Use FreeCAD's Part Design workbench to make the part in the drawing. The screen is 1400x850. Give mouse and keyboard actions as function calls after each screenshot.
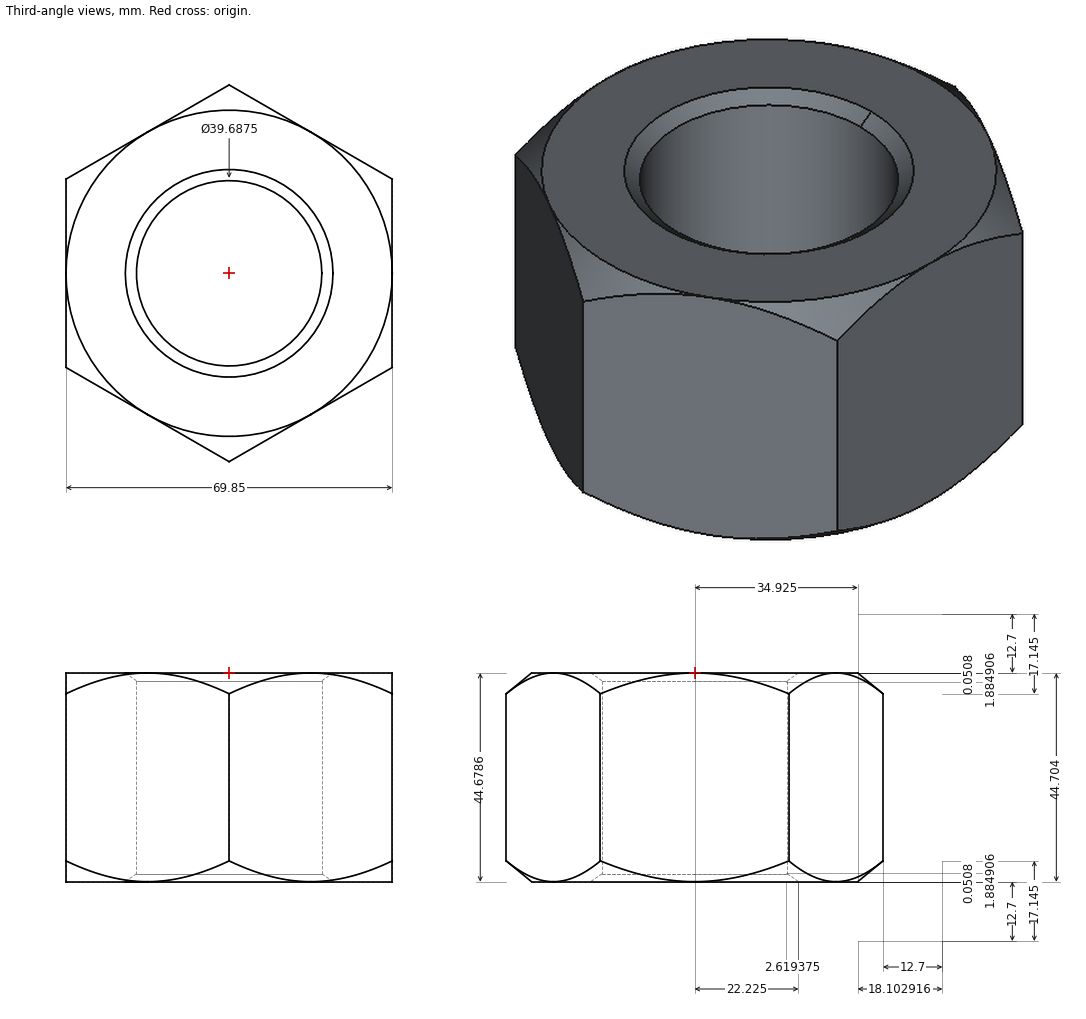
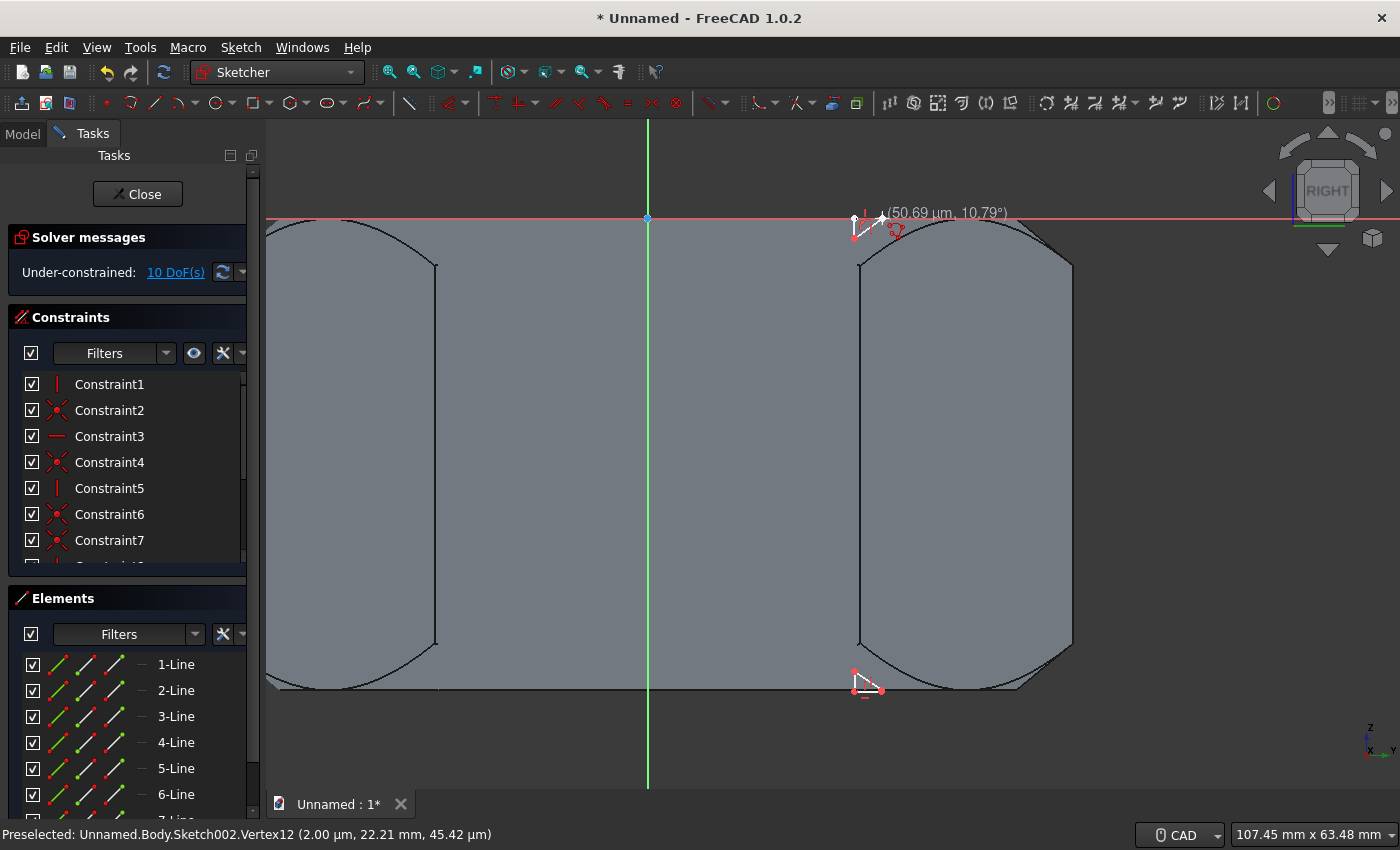
scroll(855, 218, up, 17)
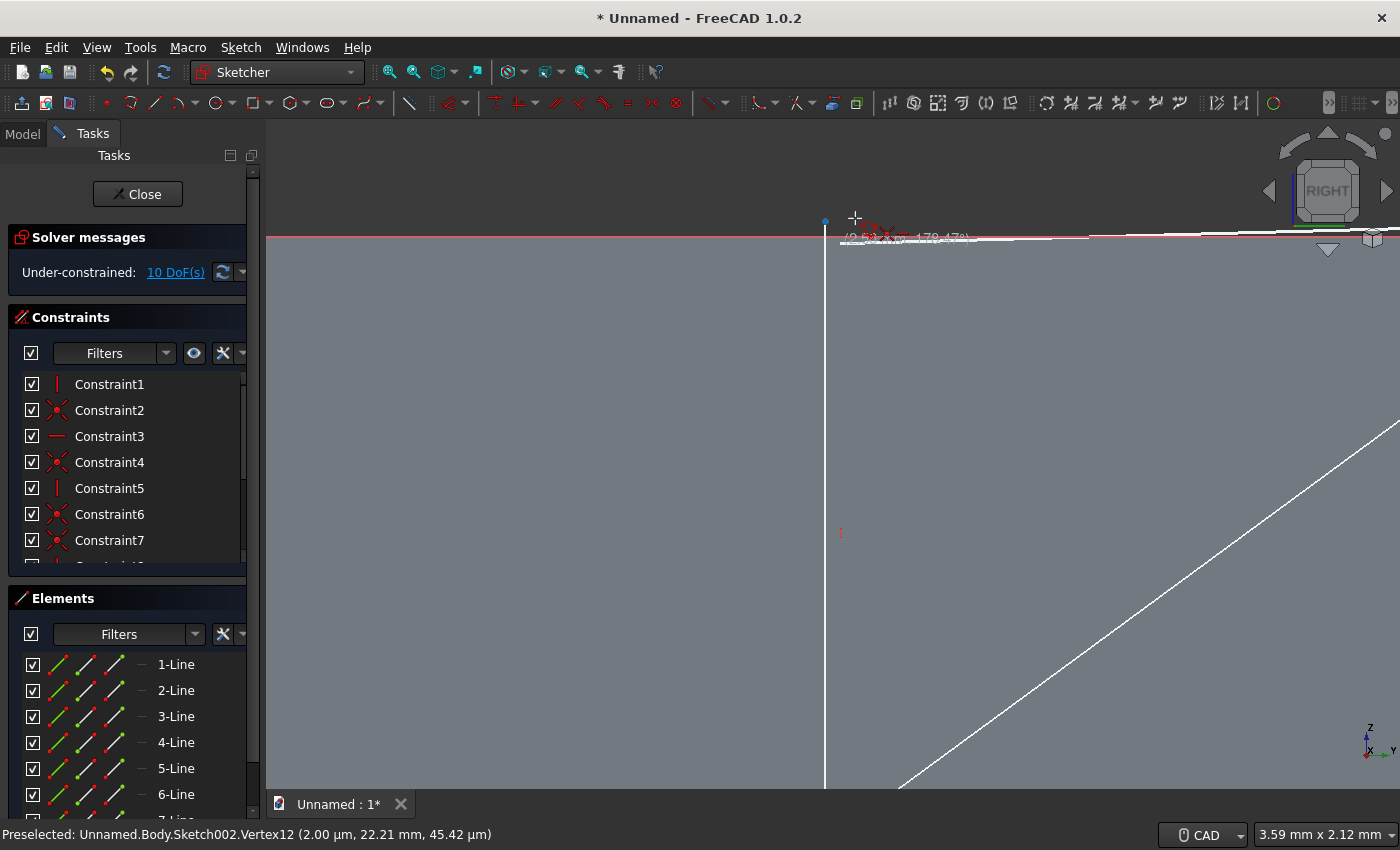
click(825, 222)
key(Escape)
key(Escape)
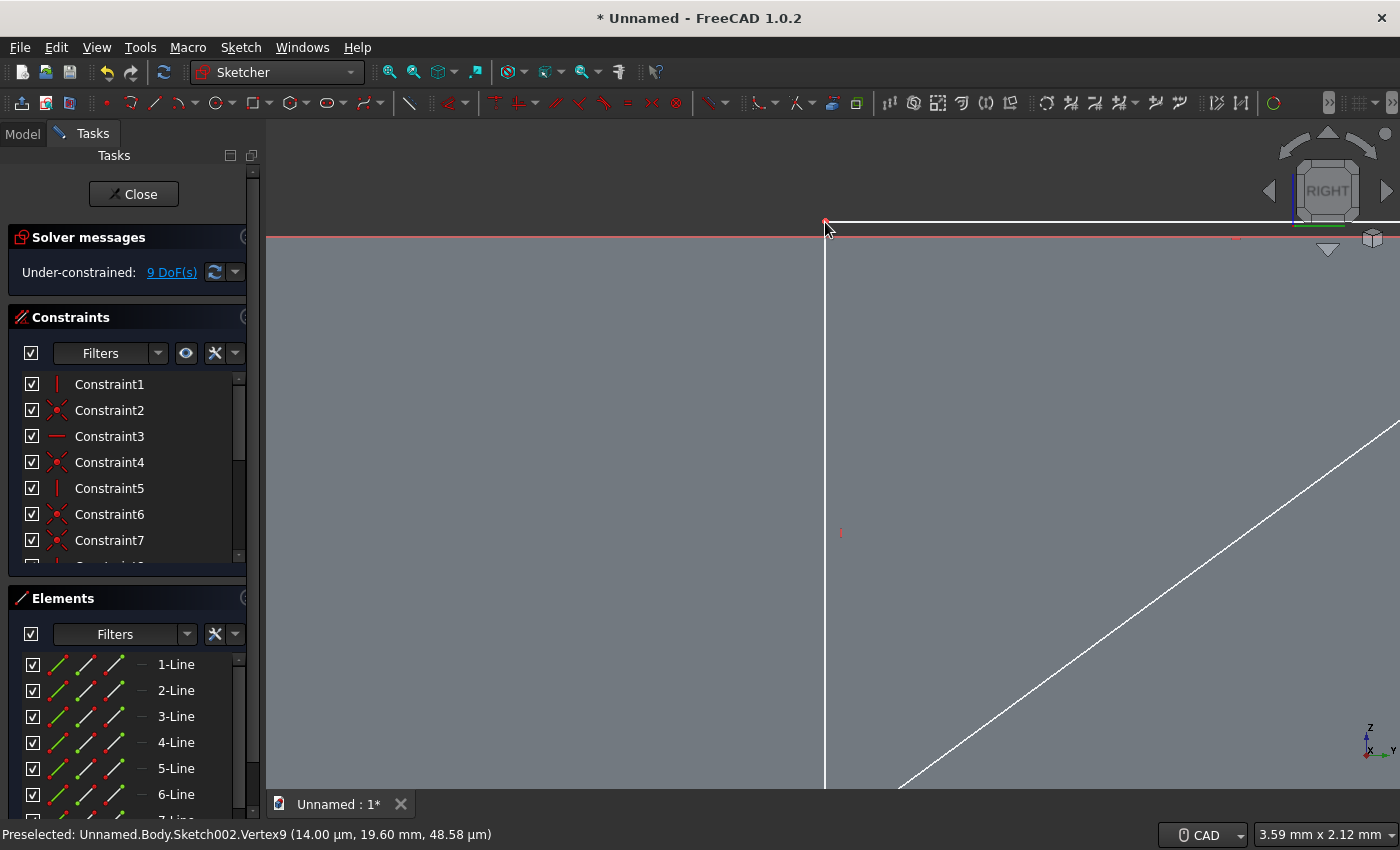
key(d)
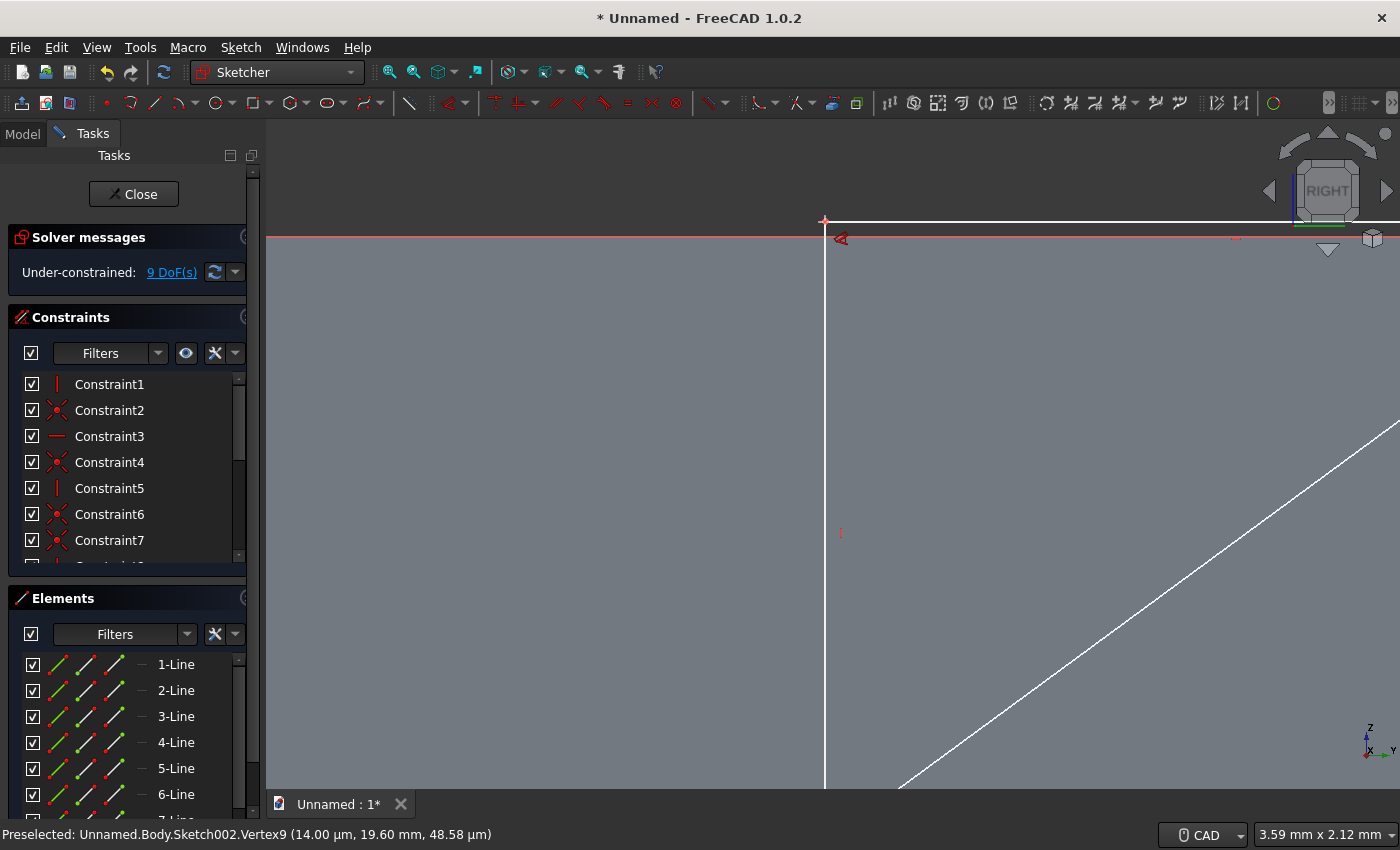
scroll(855, 218, down, 17)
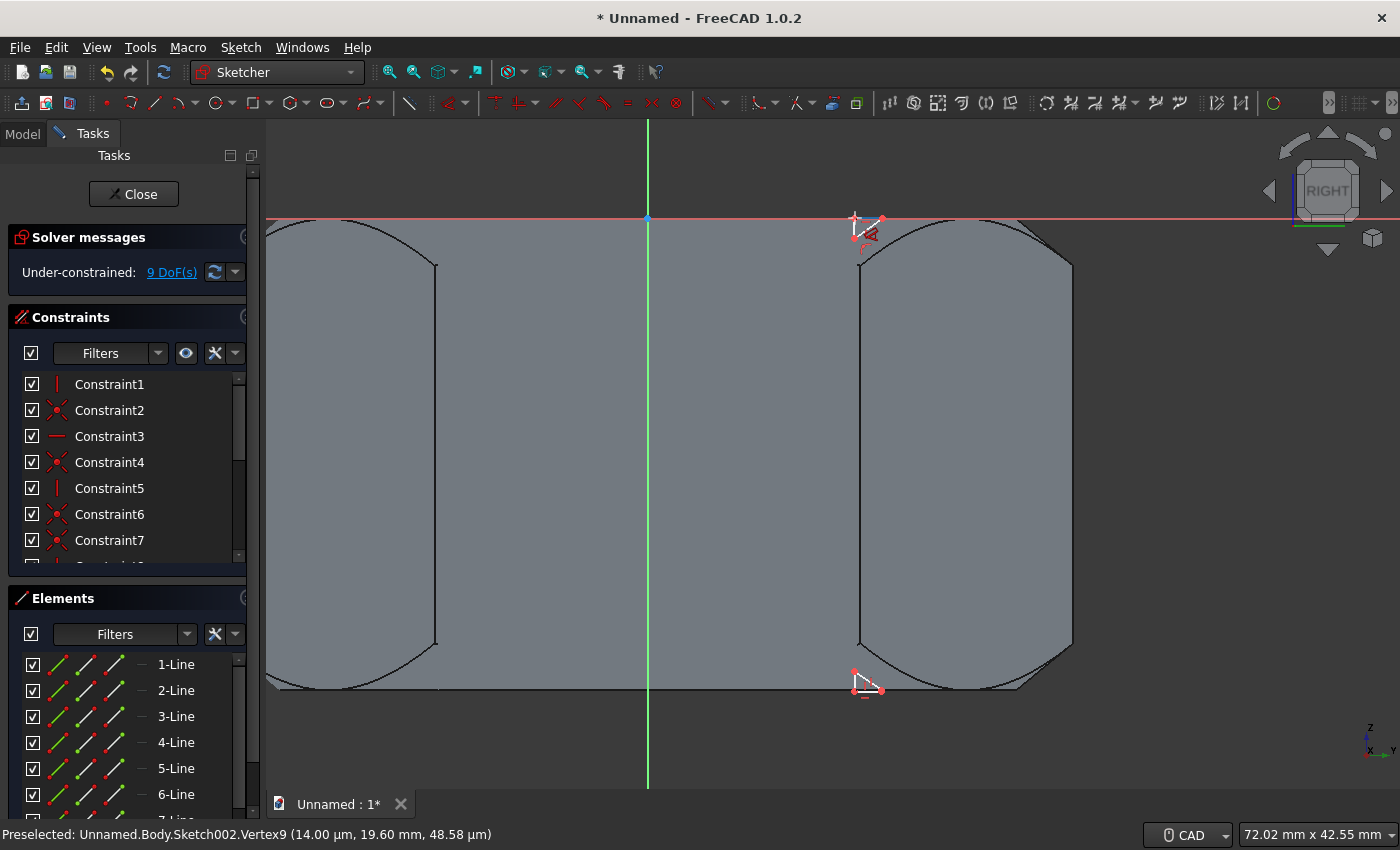
scroll(882, 691, up, 22)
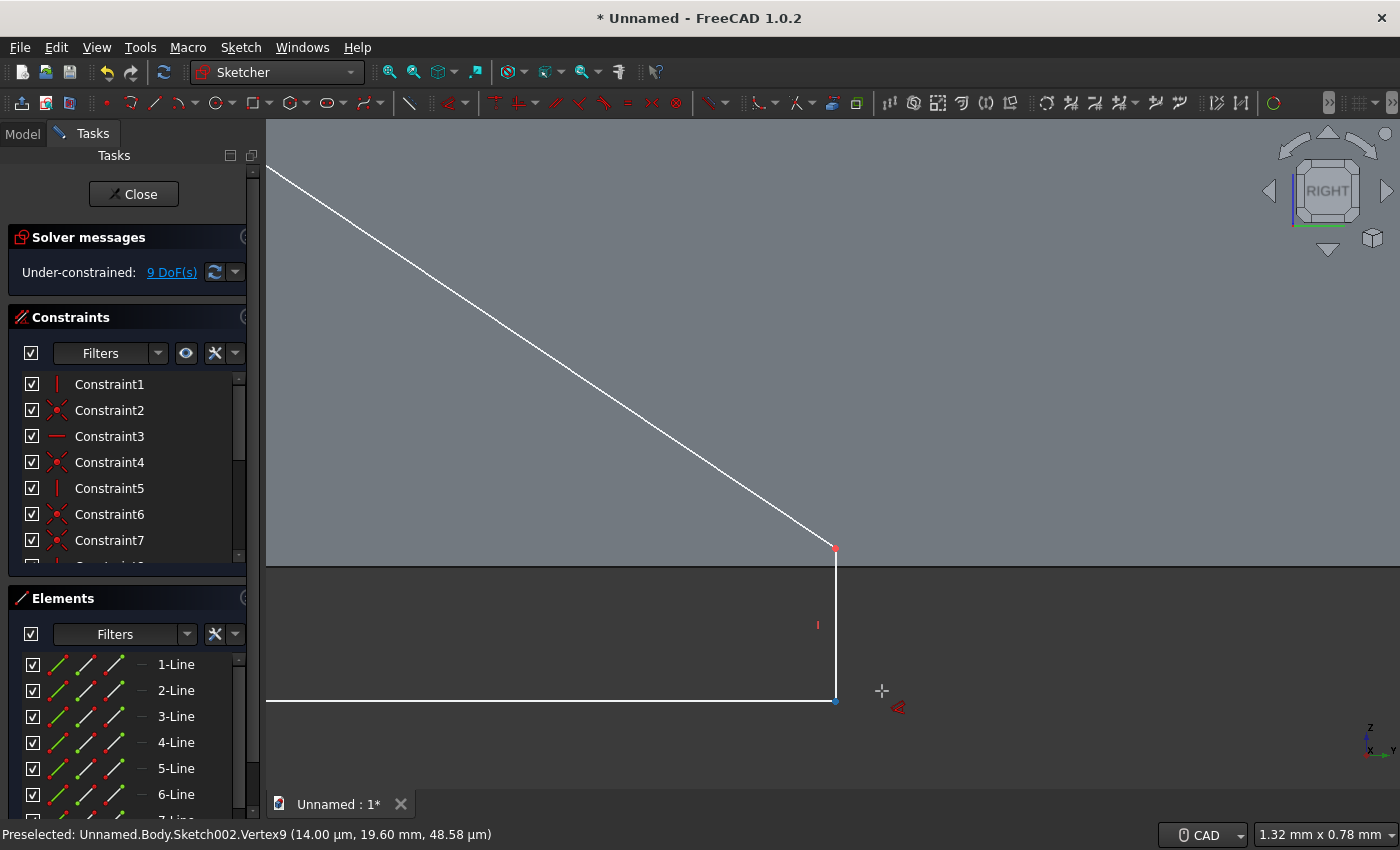
click(836, 655)
click(870, 625)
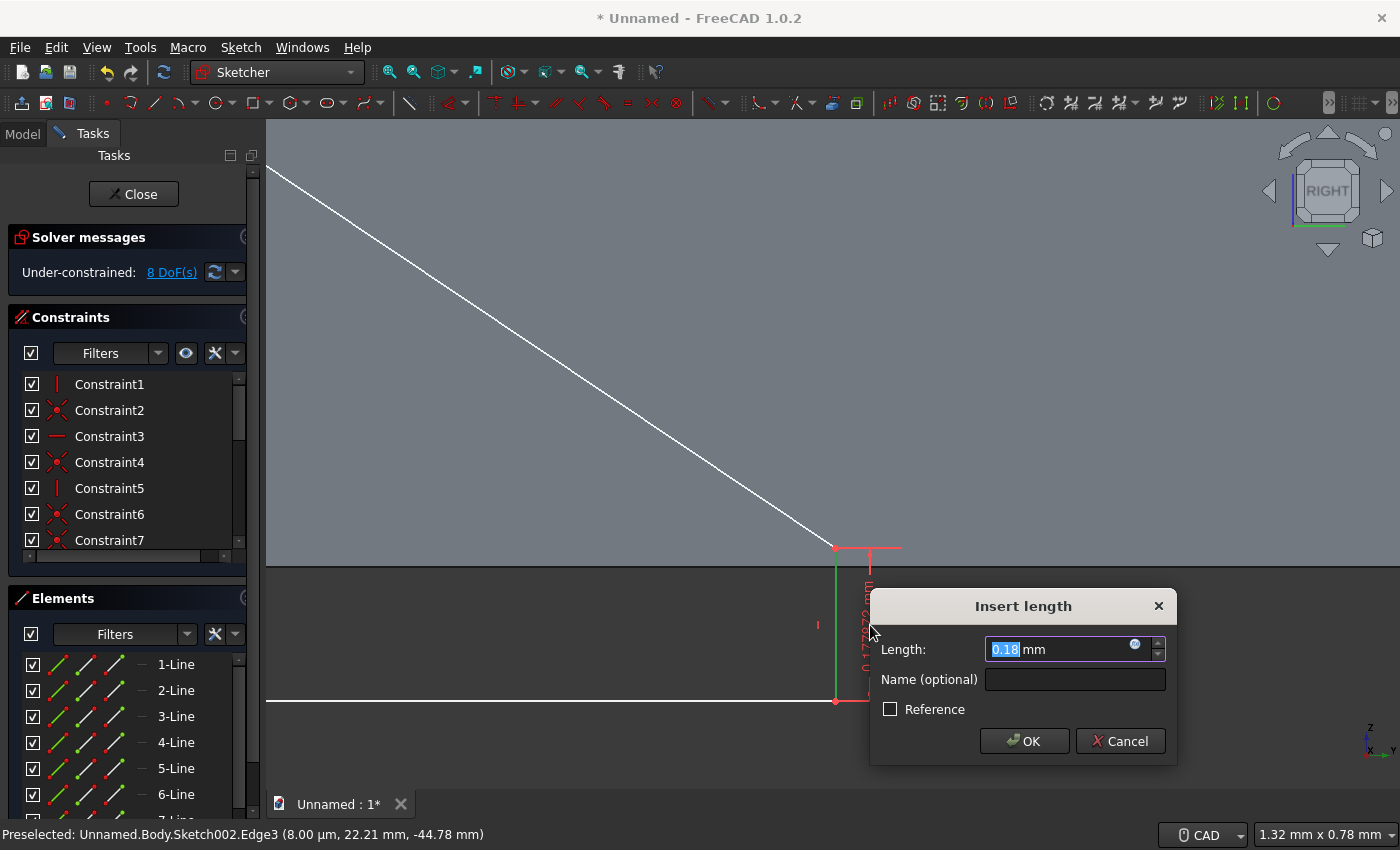
text(0.0508)
key(Return)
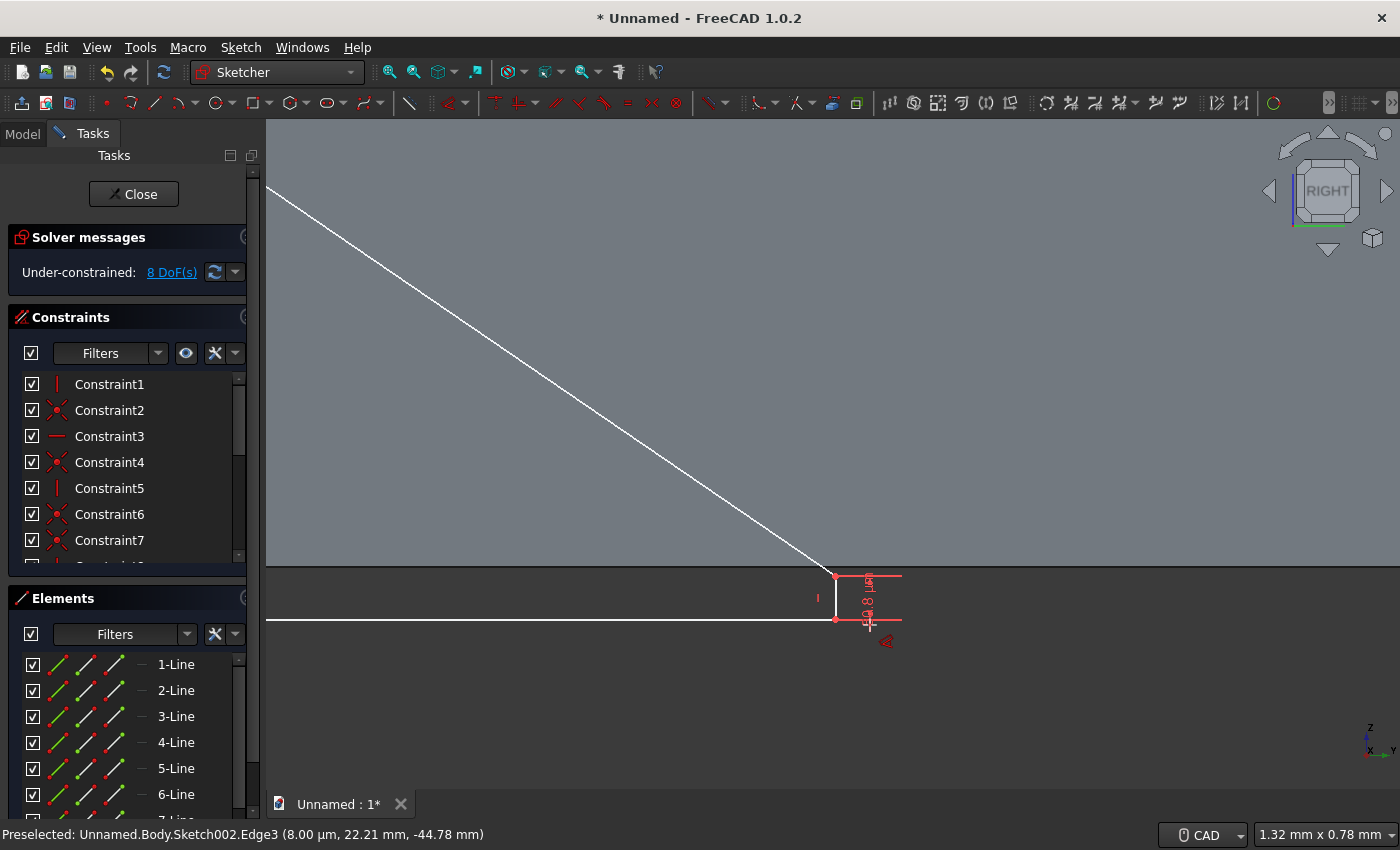
scroll(764, 454, down, 15)